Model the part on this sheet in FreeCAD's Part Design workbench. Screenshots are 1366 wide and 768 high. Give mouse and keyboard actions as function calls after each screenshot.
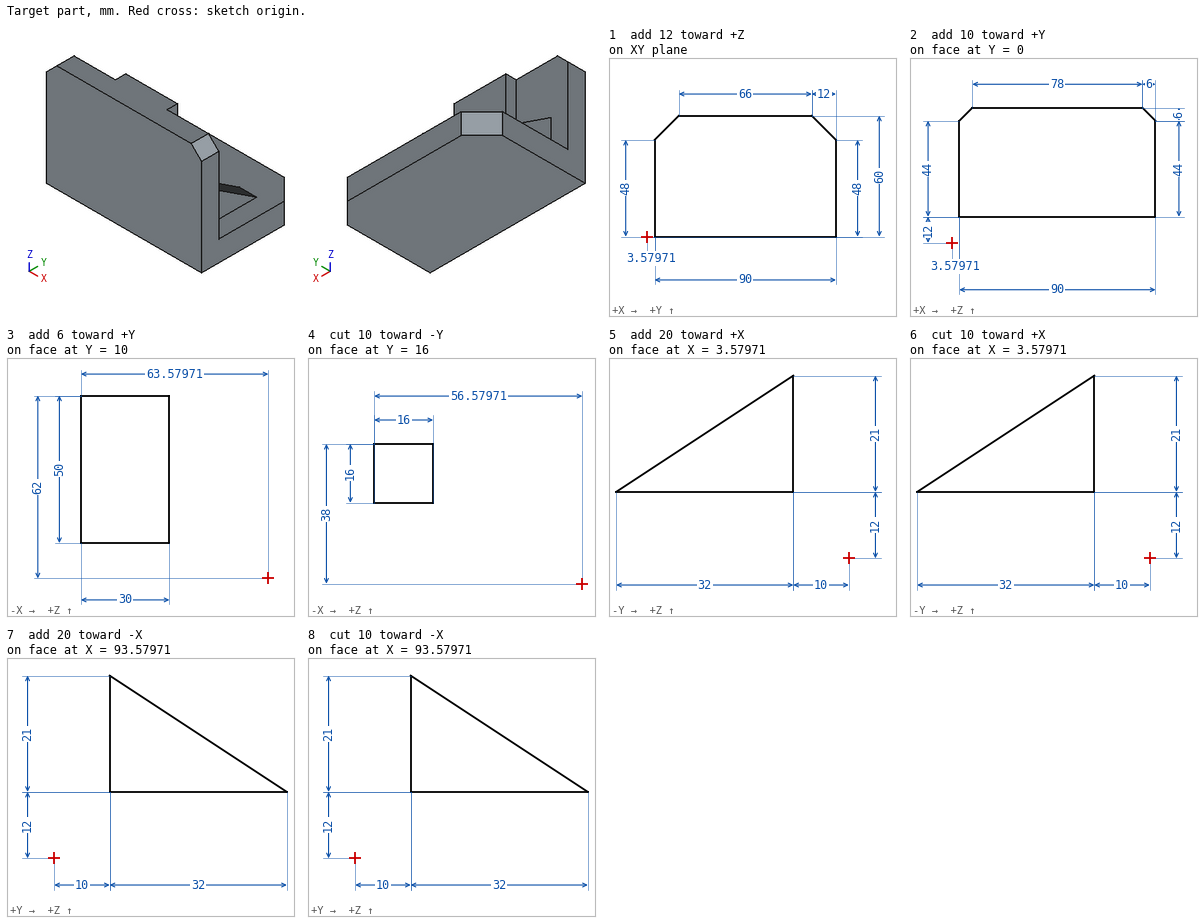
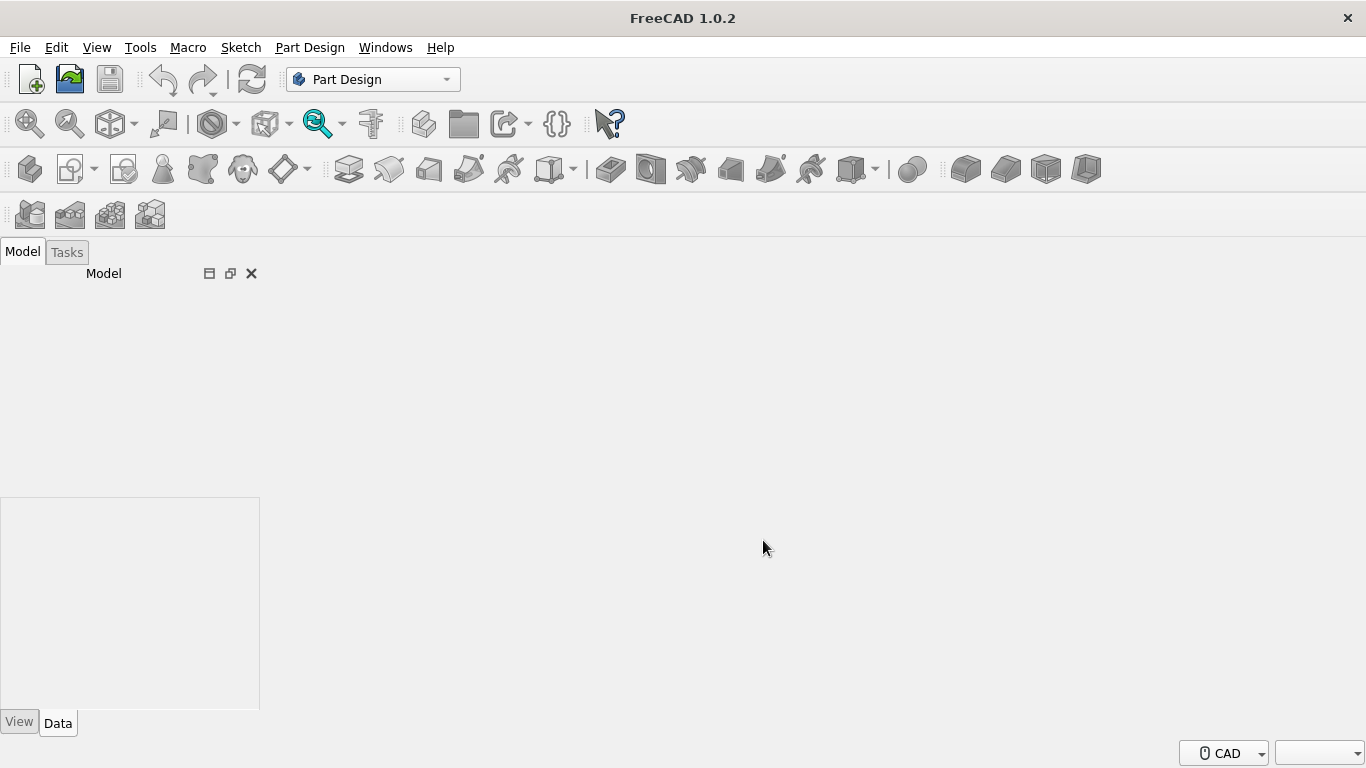
key(ctrl+n)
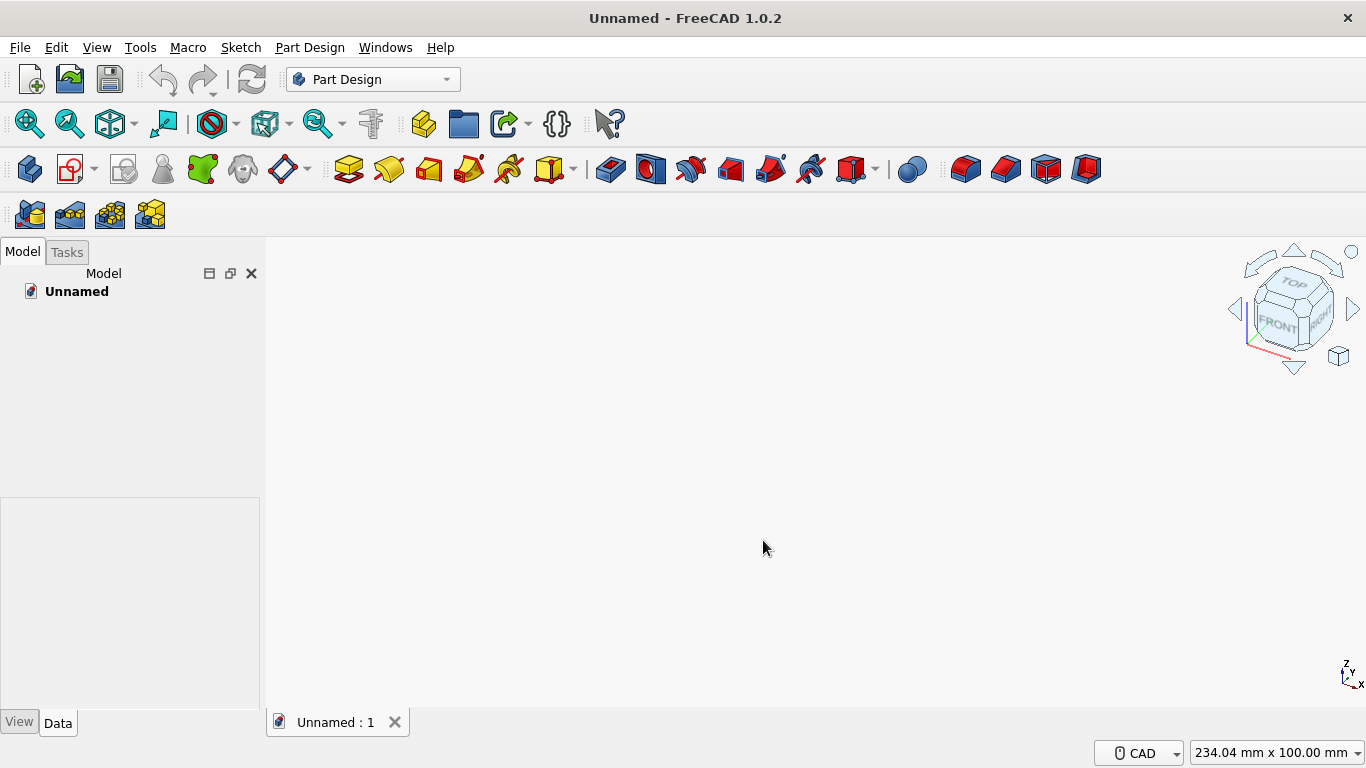
click(70, 170)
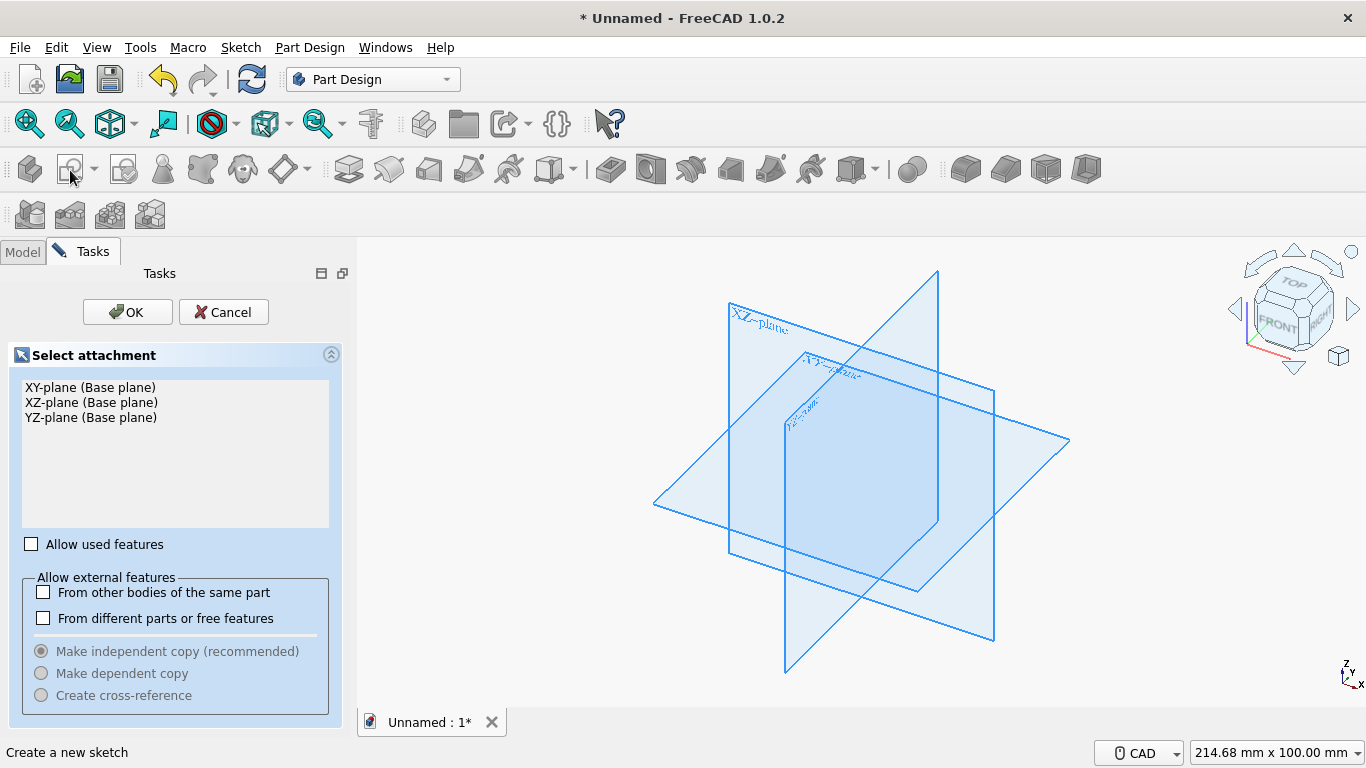
click(82, 388)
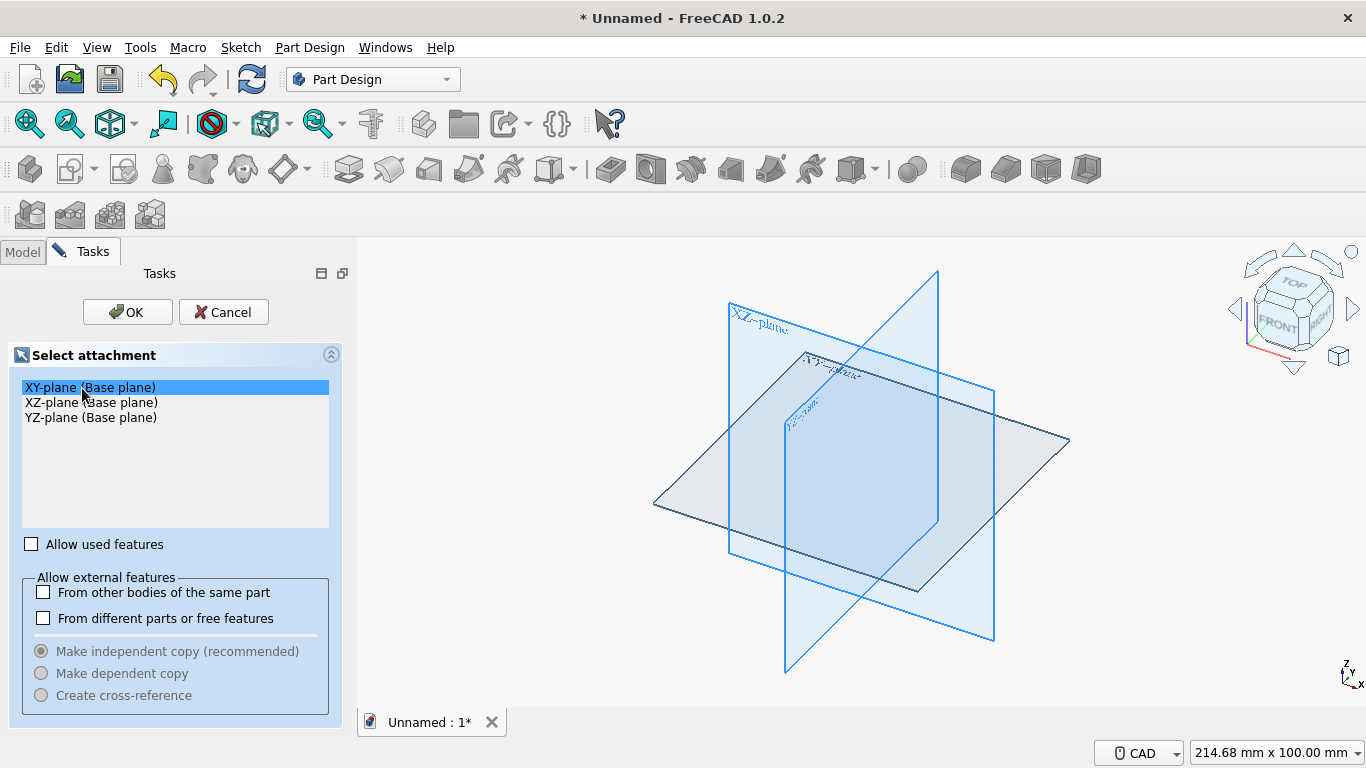
click(128, 312)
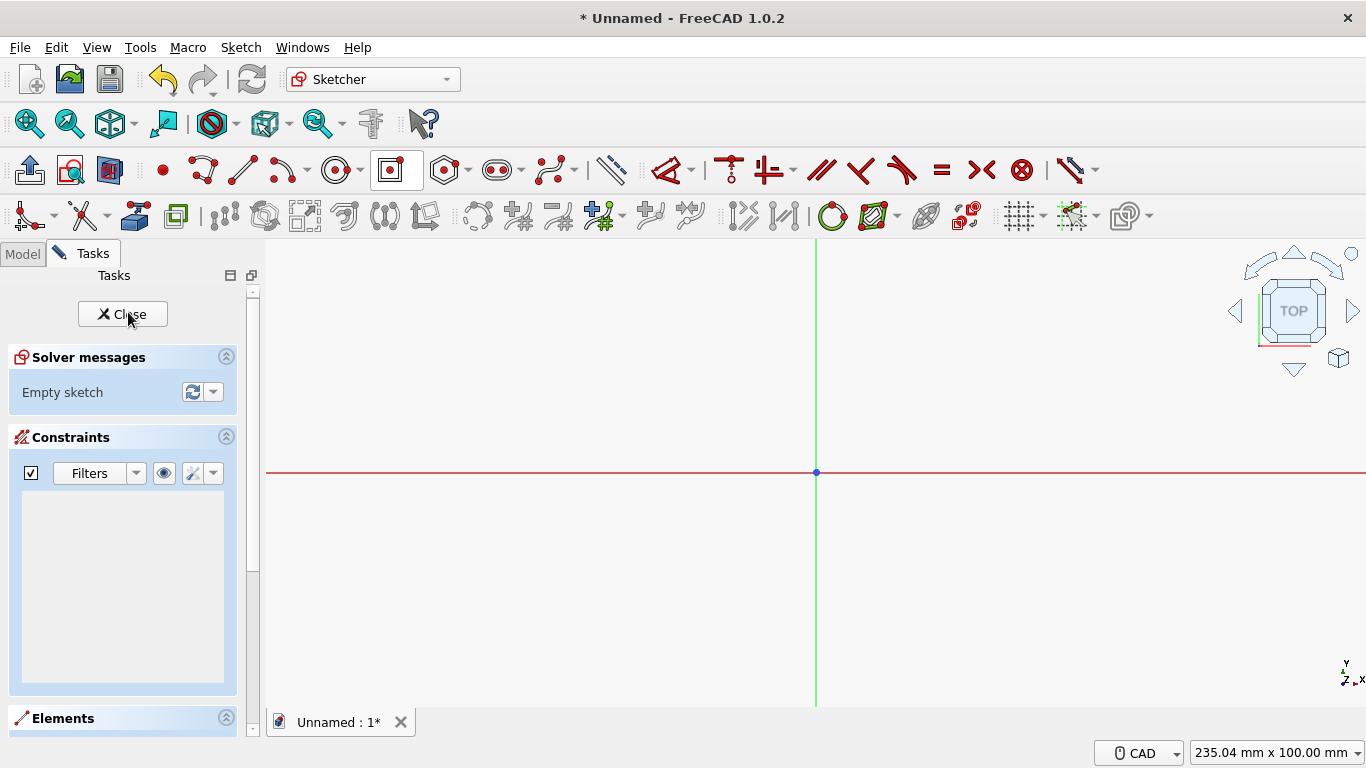
scroll(294, 679, down, 2)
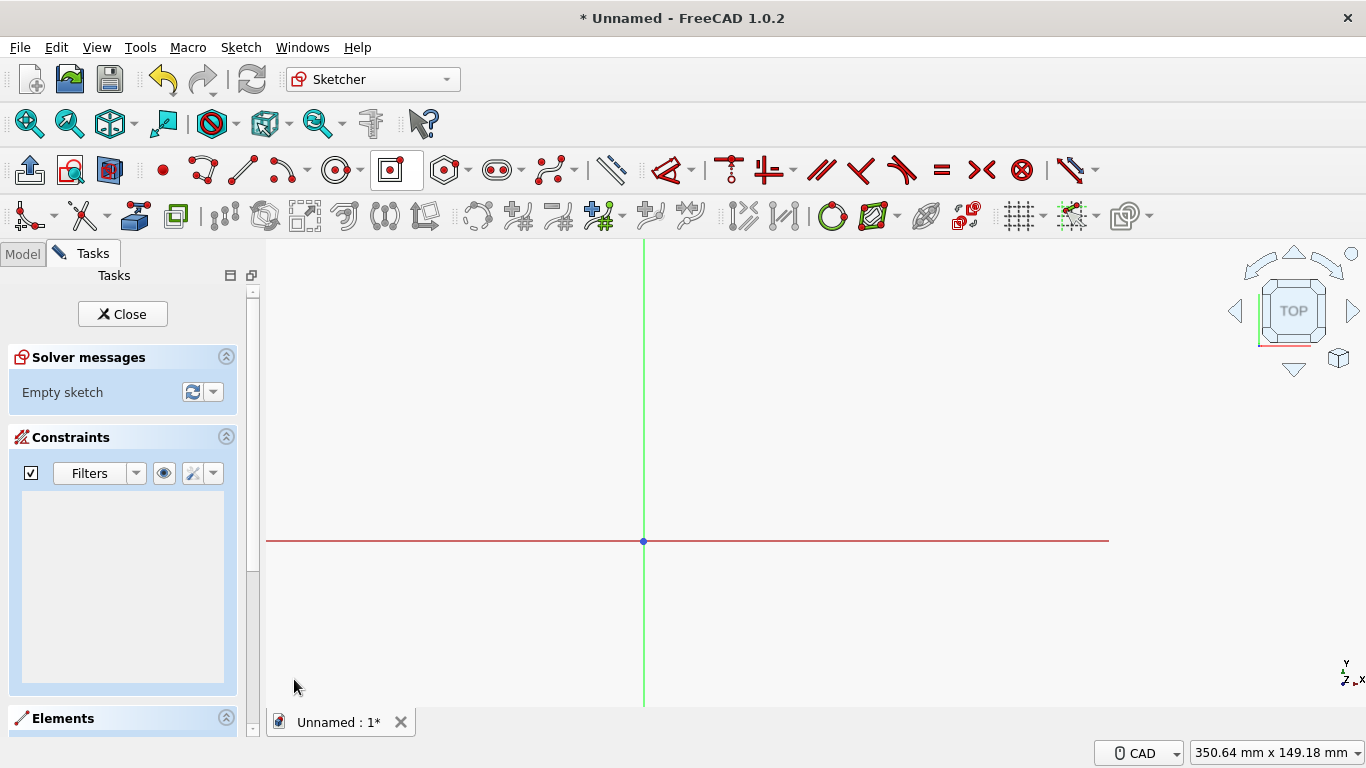
scroll(879, 394, up, 2)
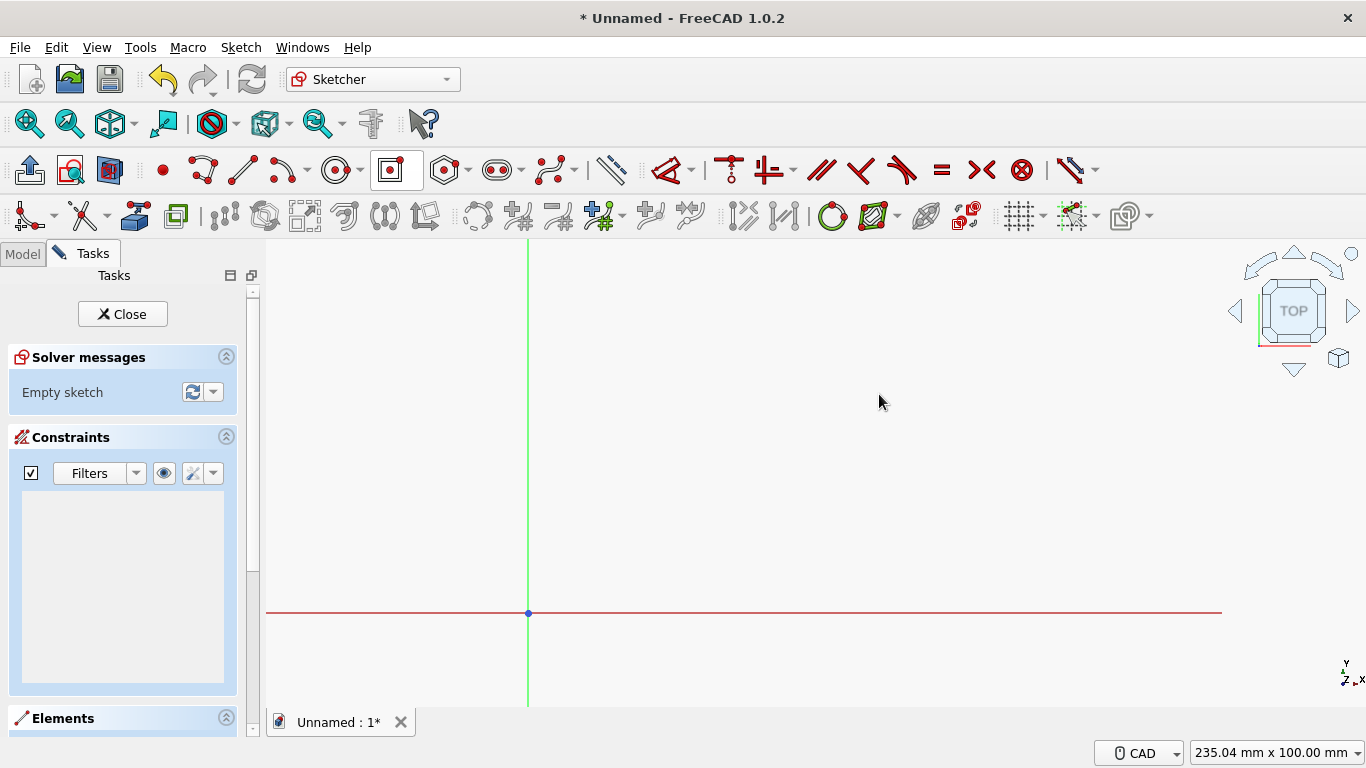
click(204, 170)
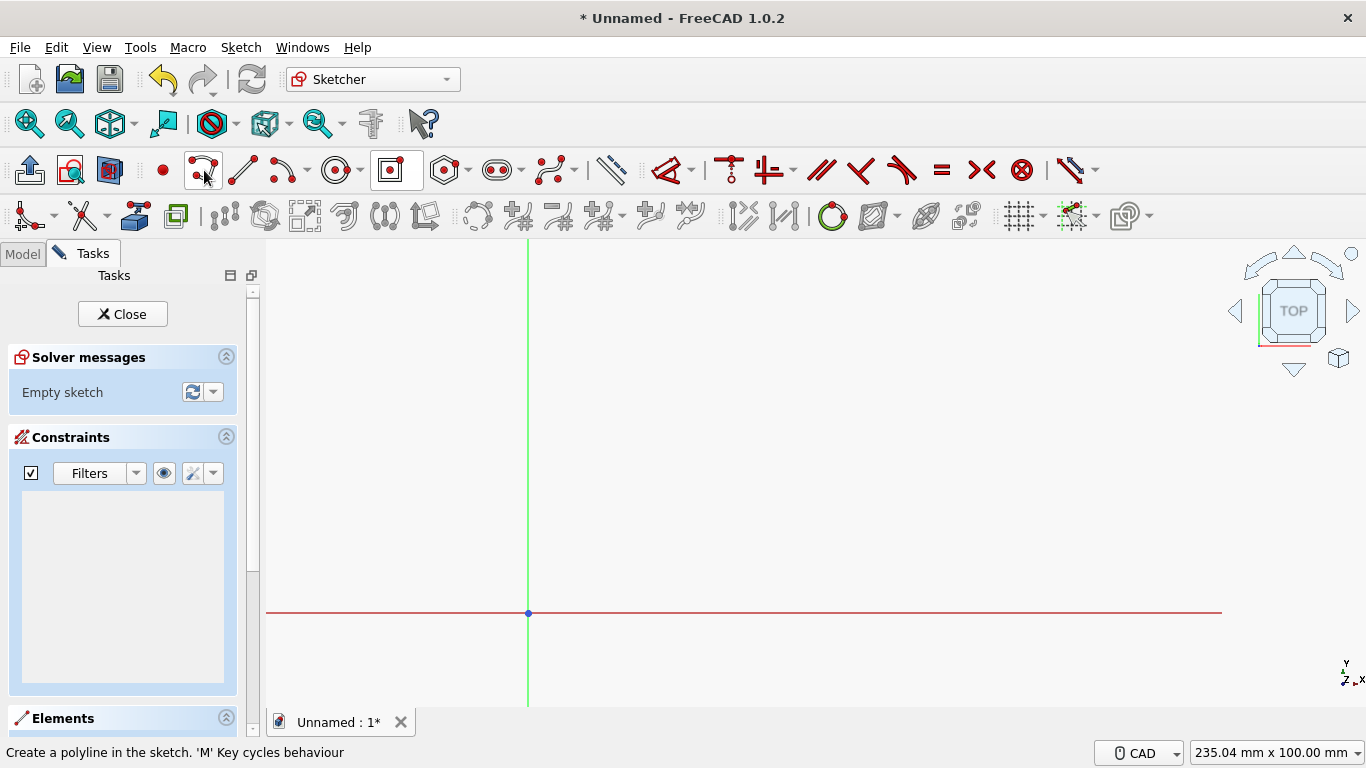
click(545, 613)
click(966, 604)
click(966, 389)
click(910, 333)
click(601, 333)
click(545, 389)
click(545, 613)
key(Escape)
key(Escape)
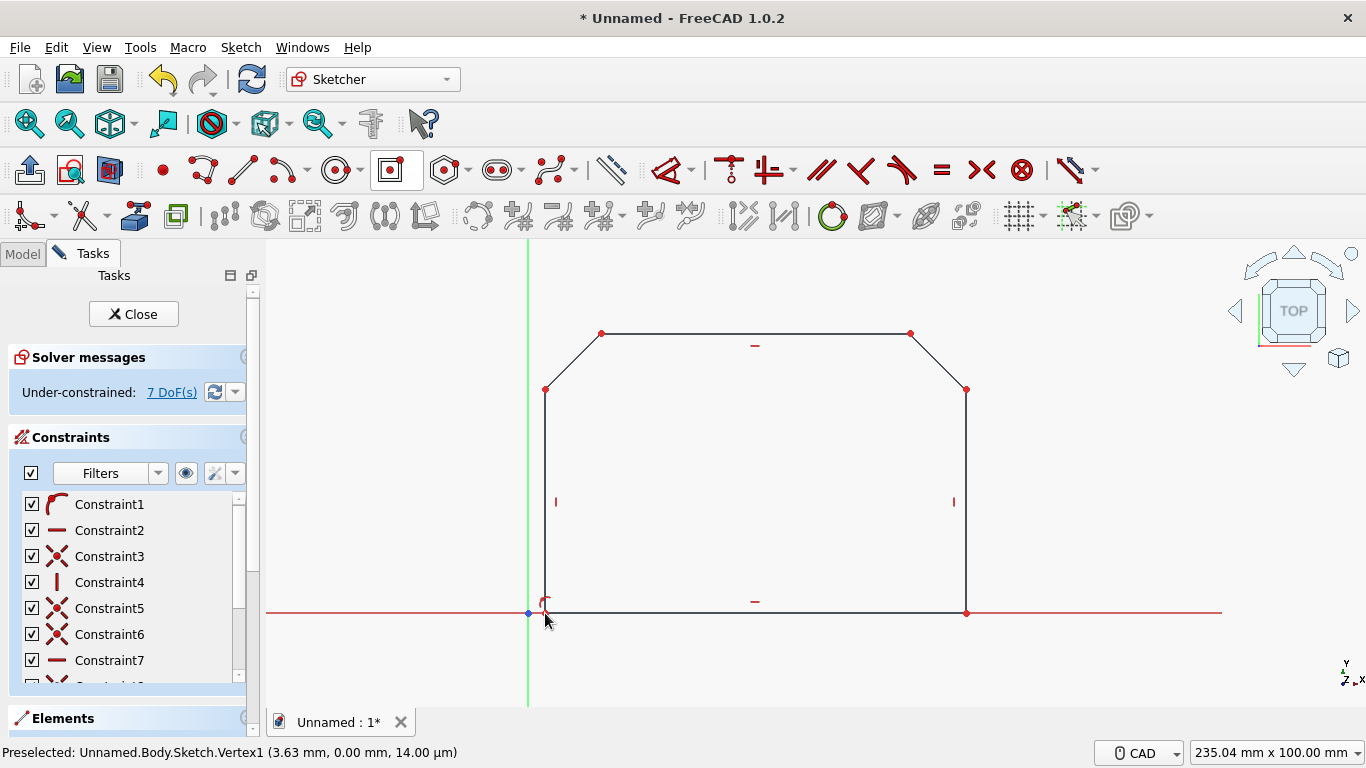
click(666, 170)